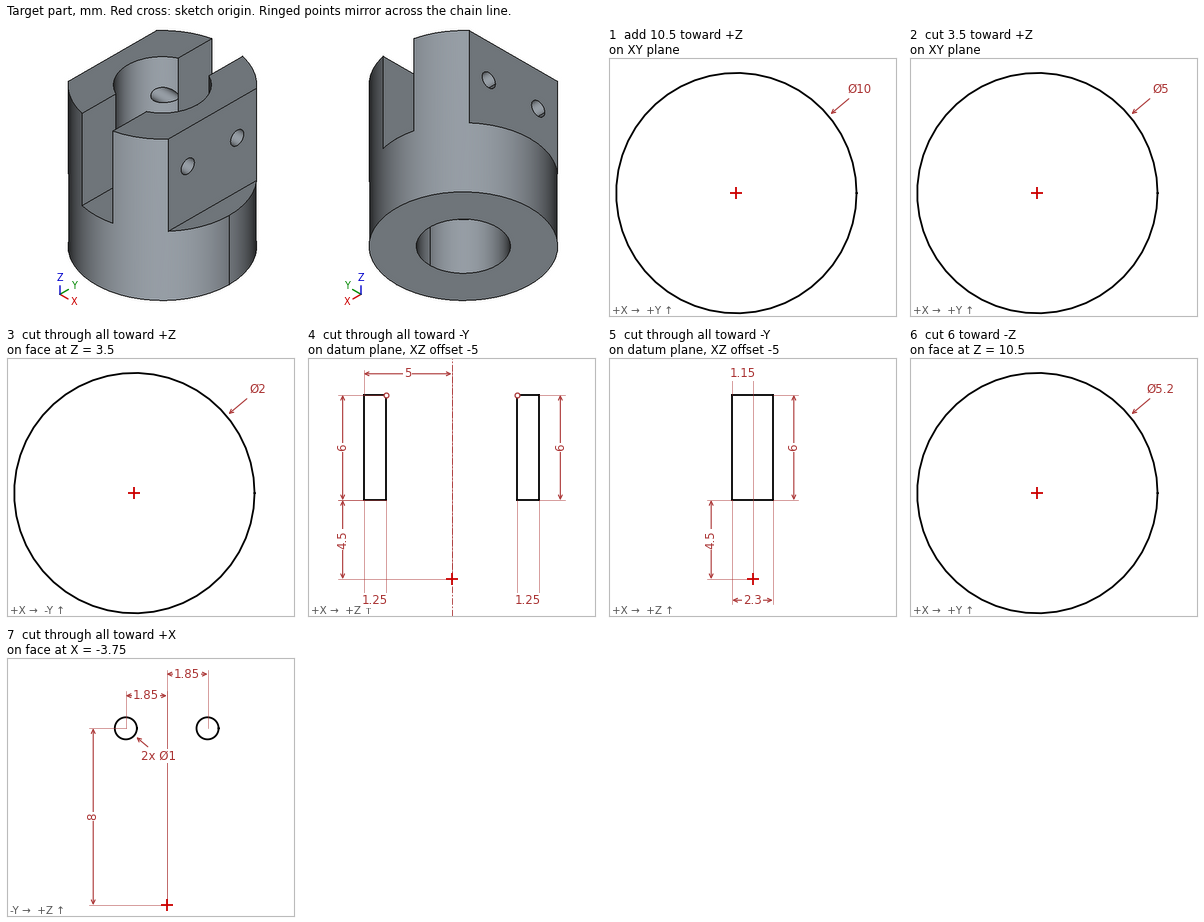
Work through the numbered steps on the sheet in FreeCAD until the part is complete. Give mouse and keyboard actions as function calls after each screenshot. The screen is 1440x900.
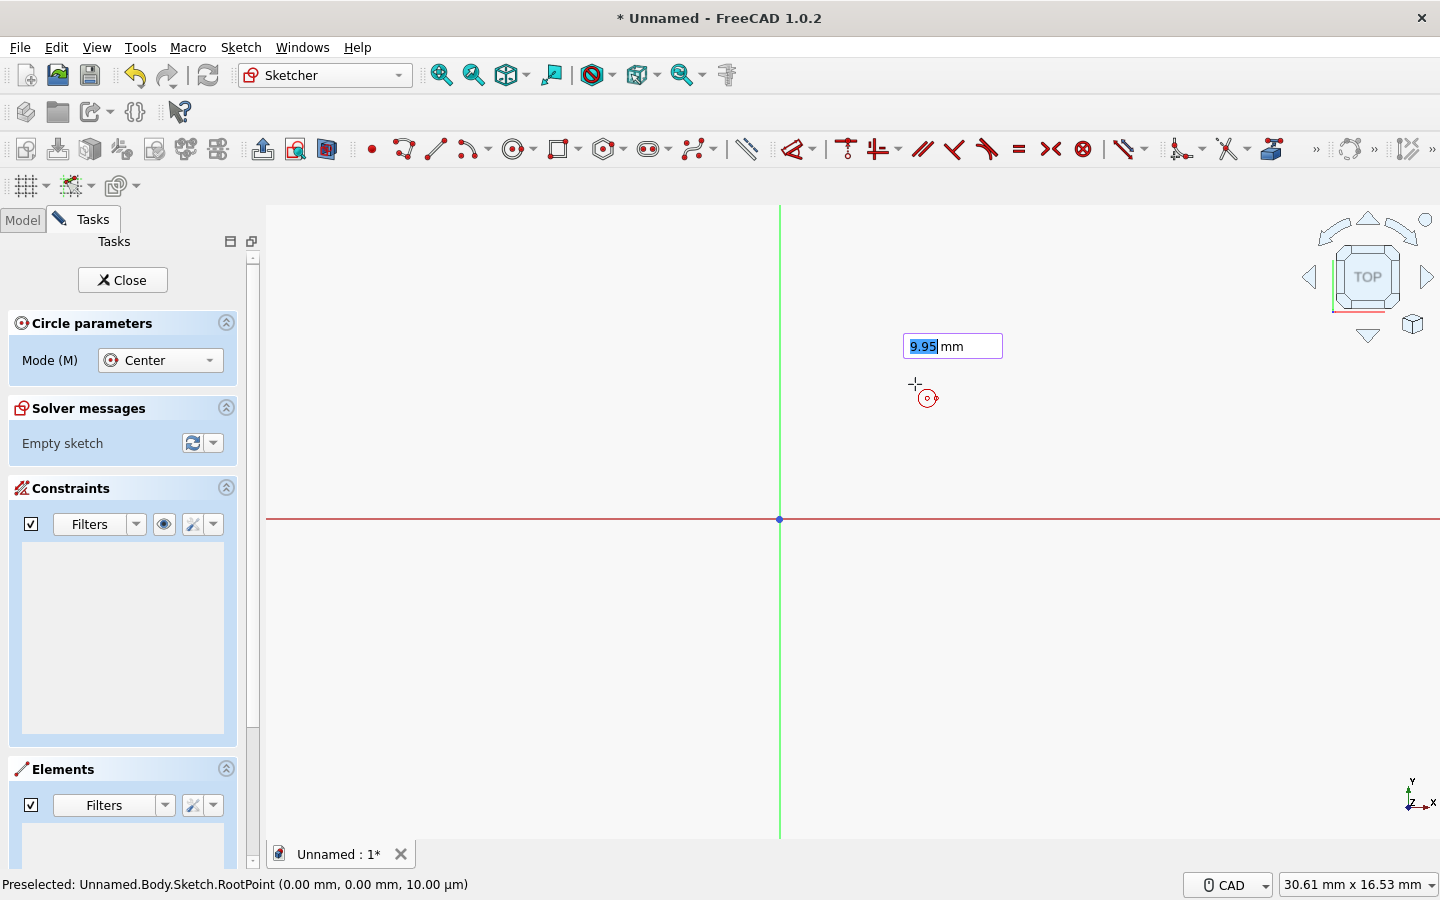
text(10)
key(Return)
key(Escape)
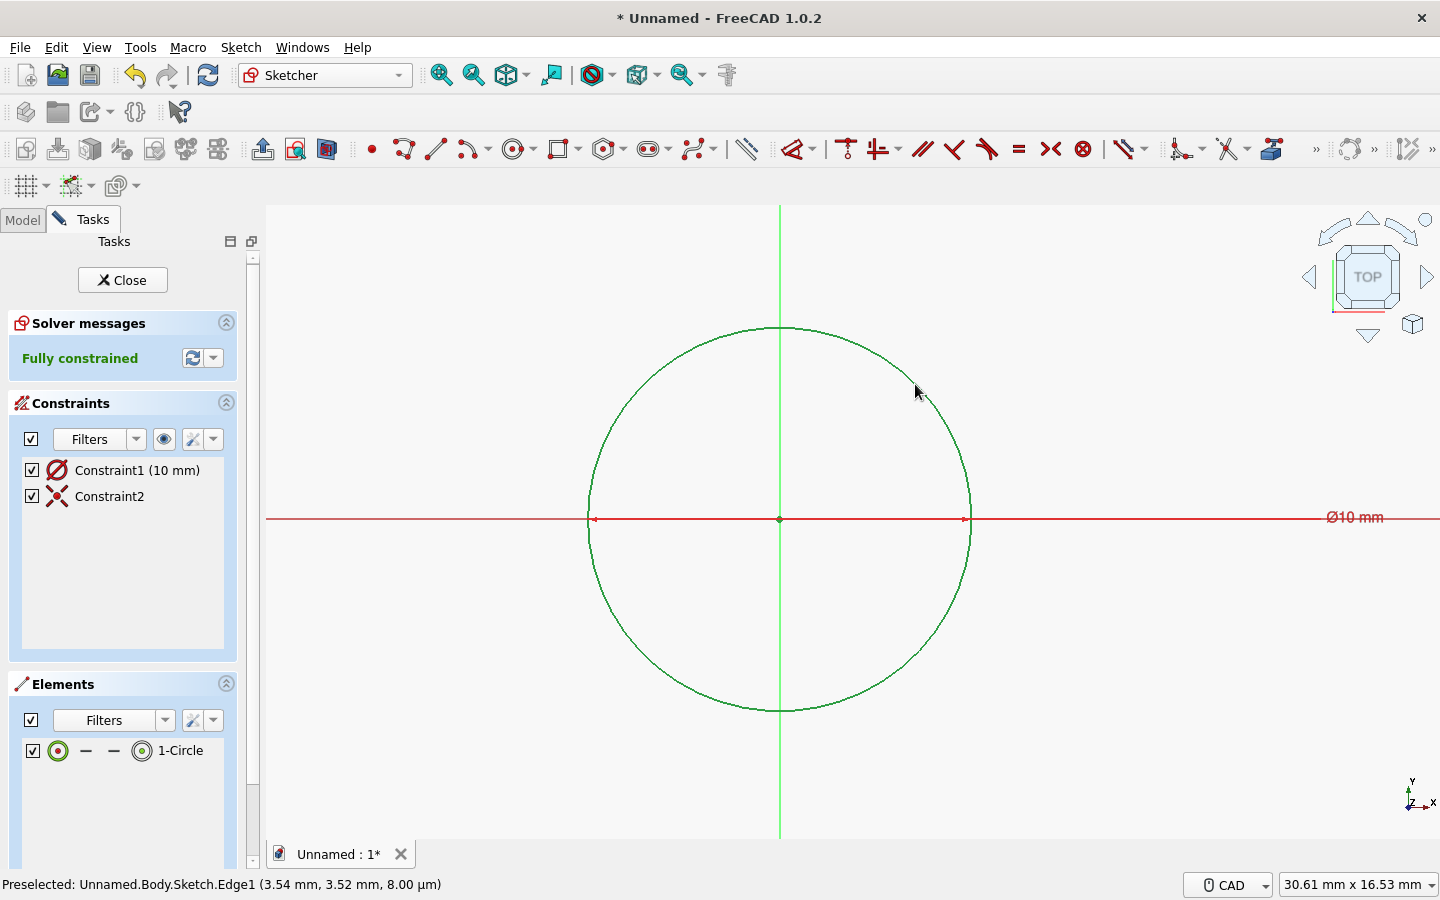
click(123, 280)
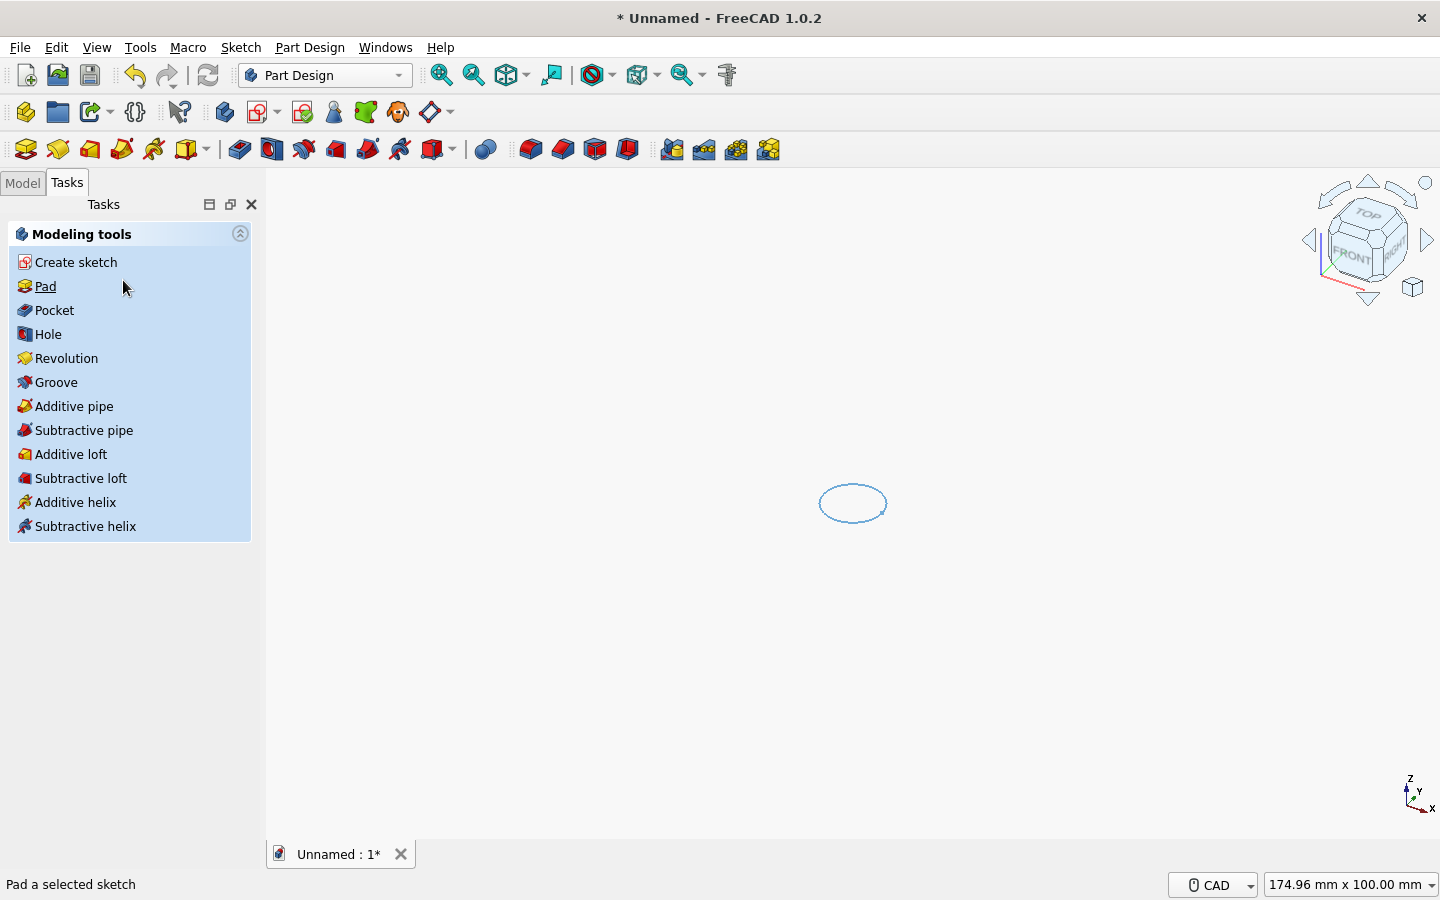
click(26, 150)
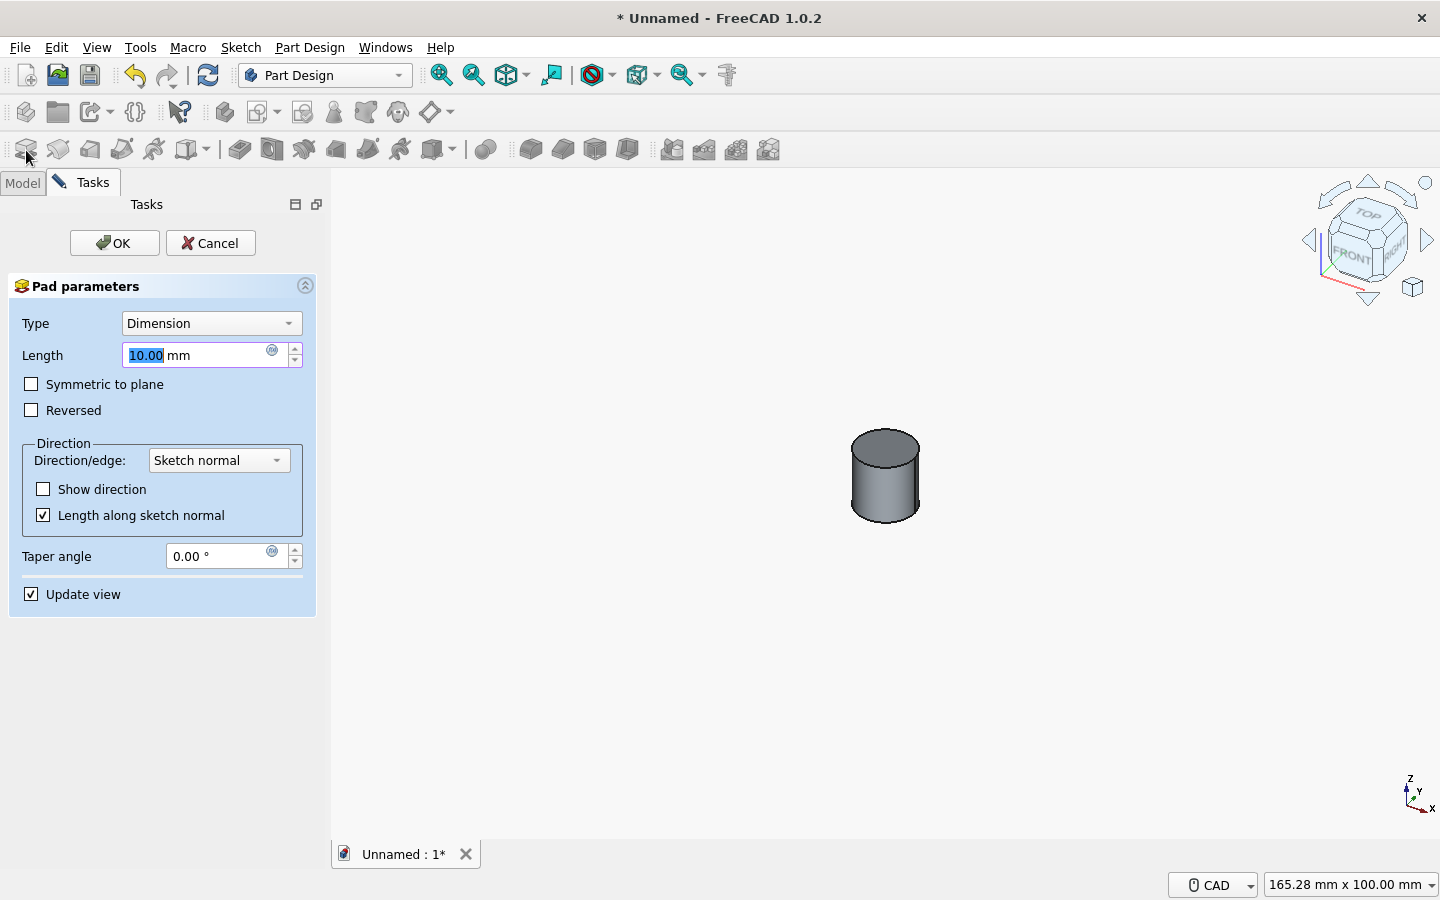
text(10.5)
key(Tab)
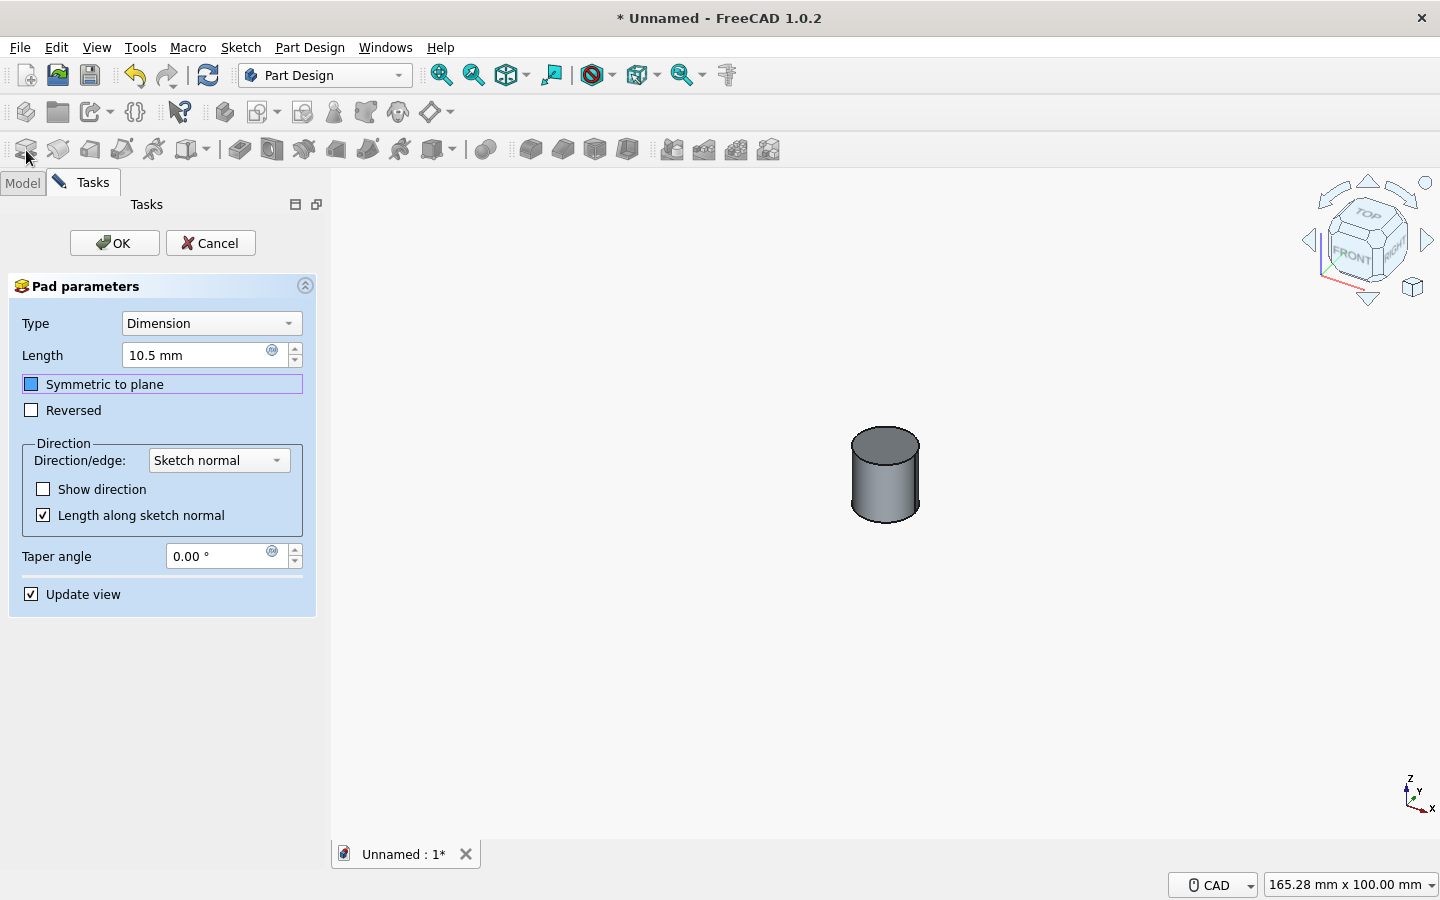
click(115, 243)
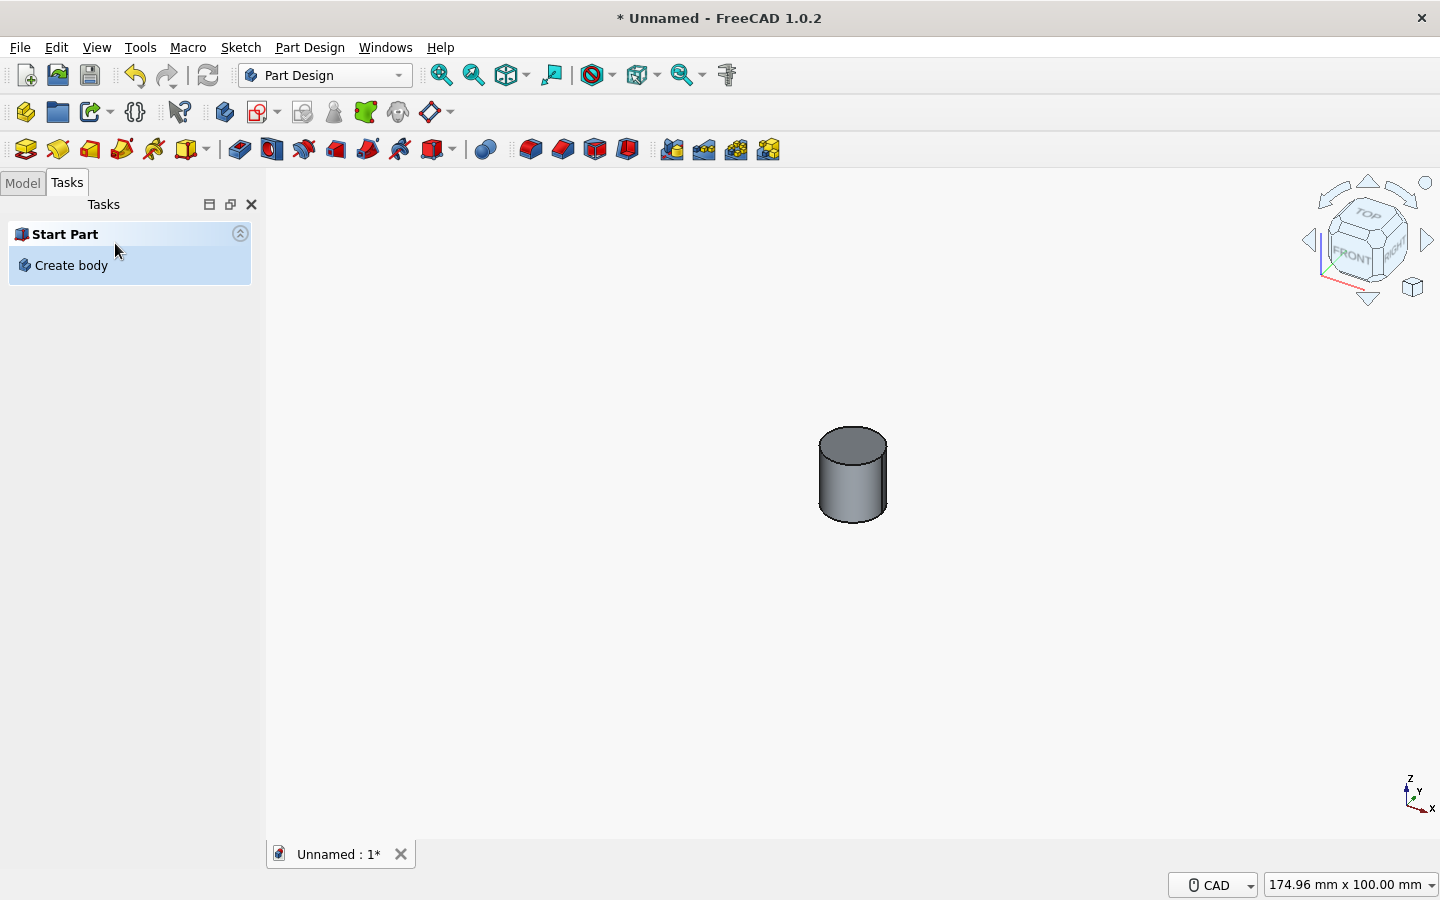
key(v)
key(f)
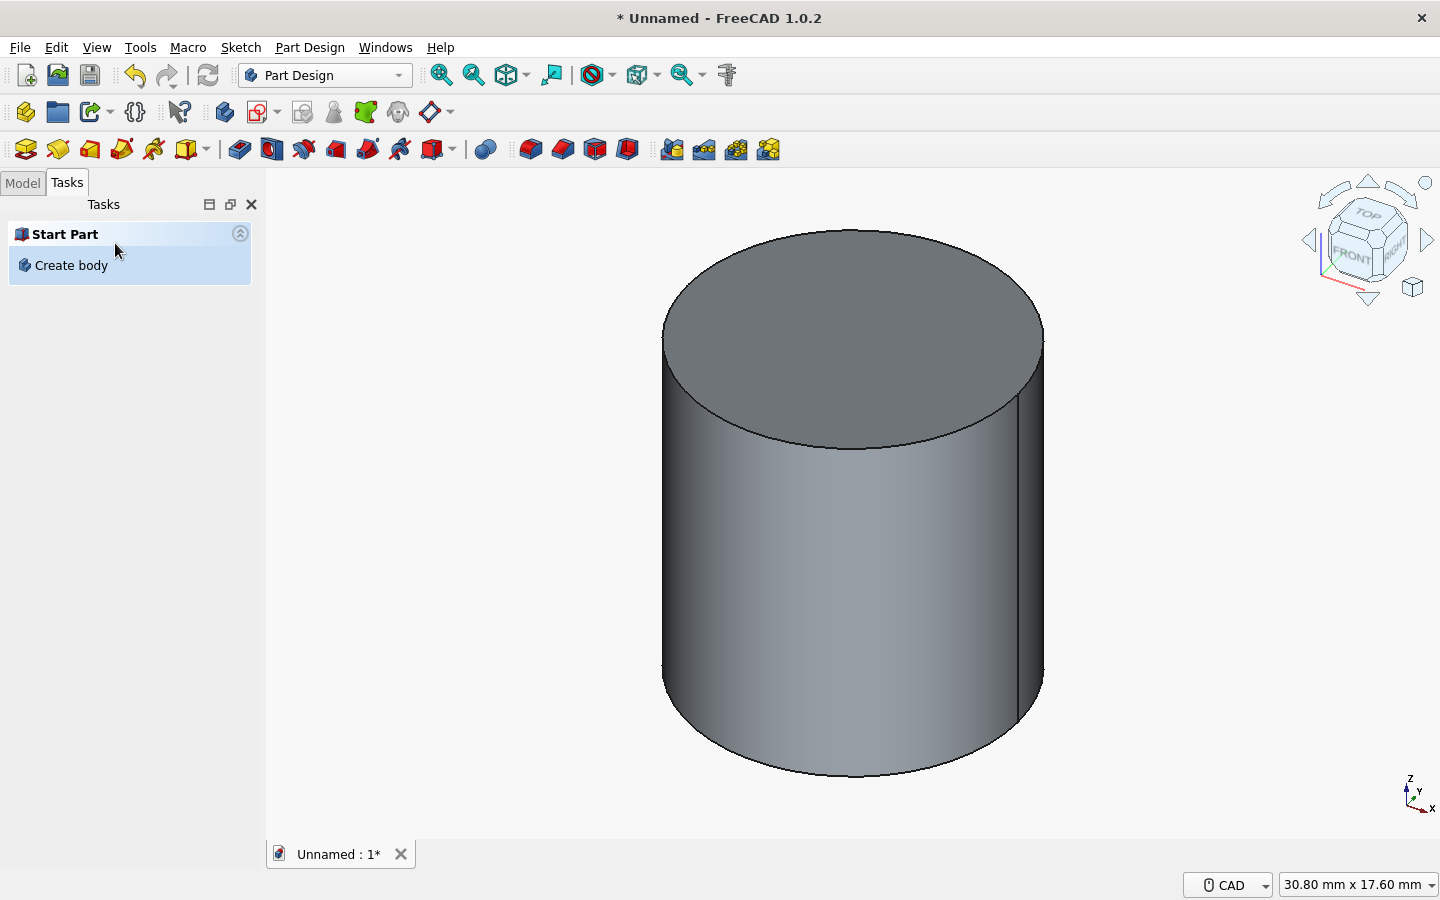
click(258, 112)